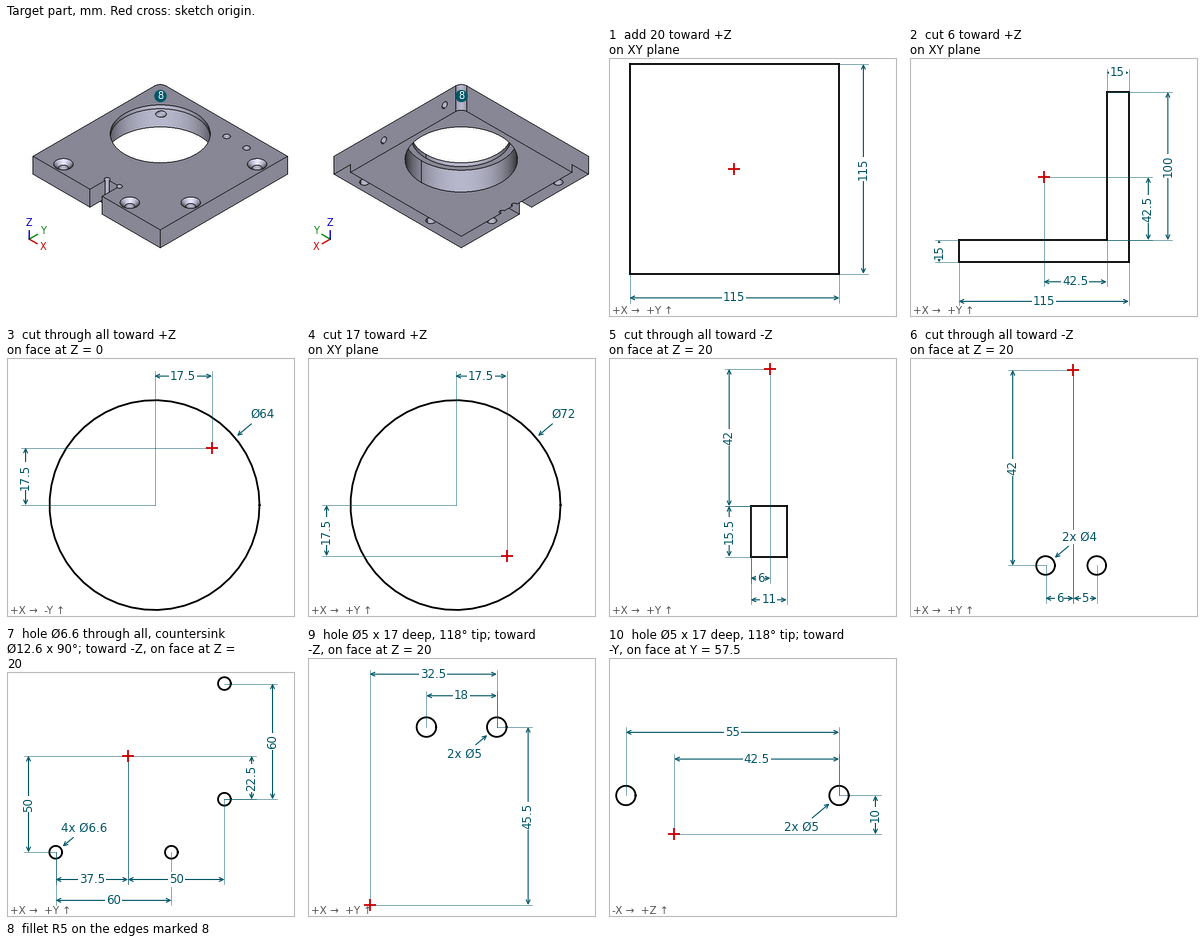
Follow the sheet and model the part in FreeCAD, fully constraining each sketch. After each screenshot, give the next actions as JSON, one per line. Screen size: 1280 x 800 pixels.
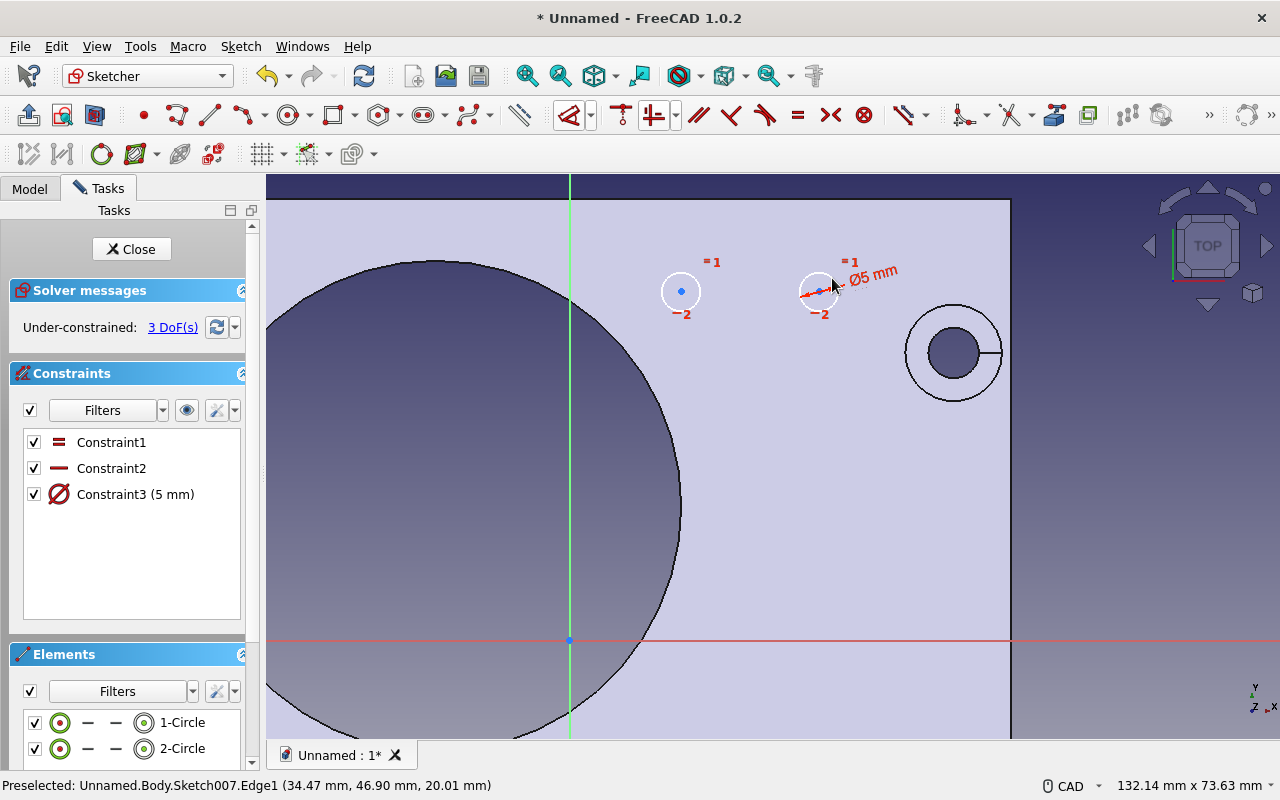
{"action": "left_click", "coordinate": [819, 292]}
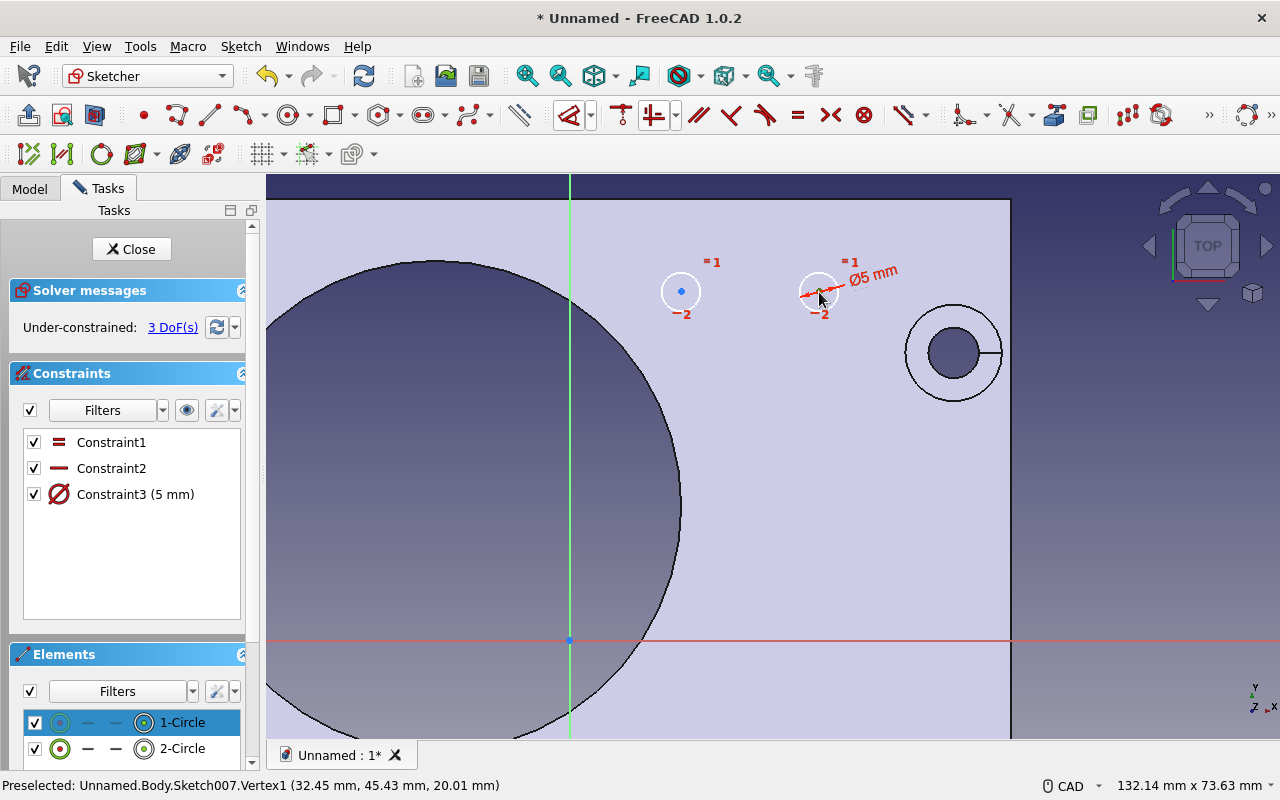
{"action": "left_click", "coordinate": [681, 292]}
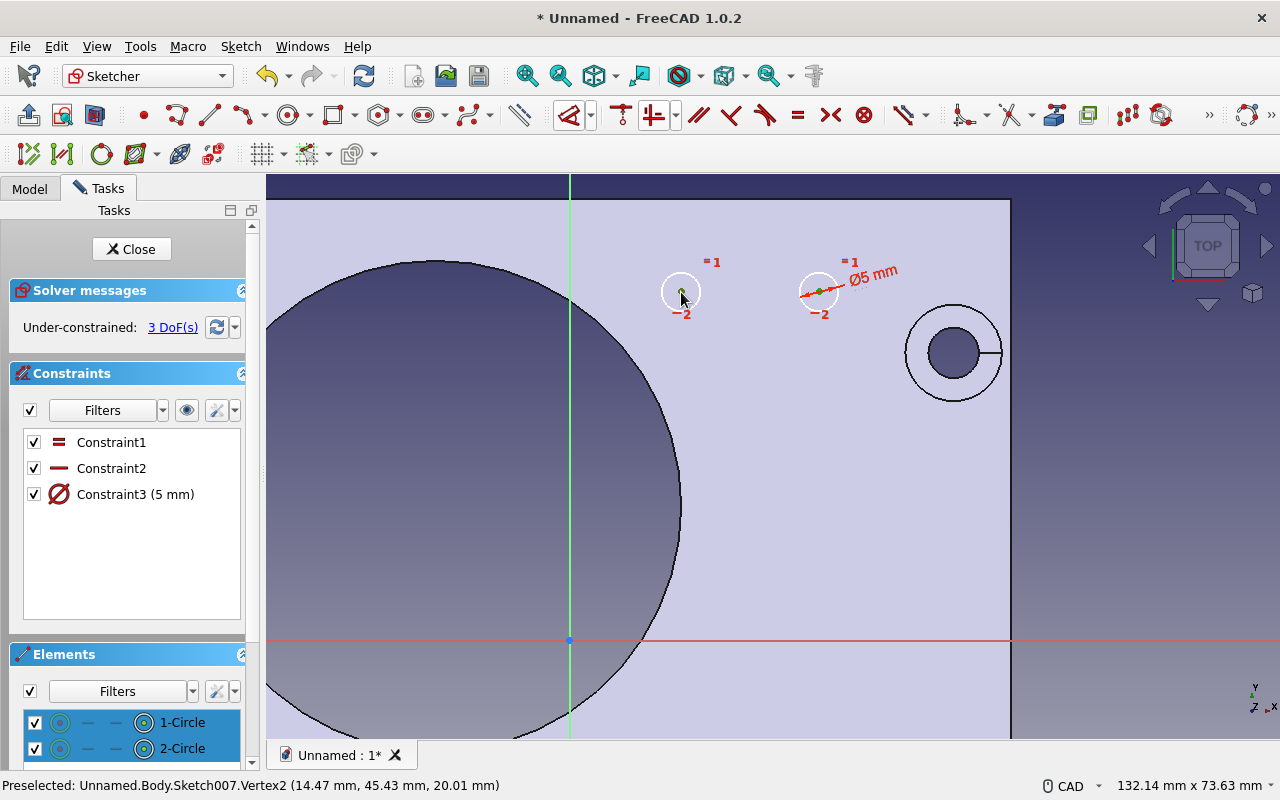
{"action": "key", "text": "l"}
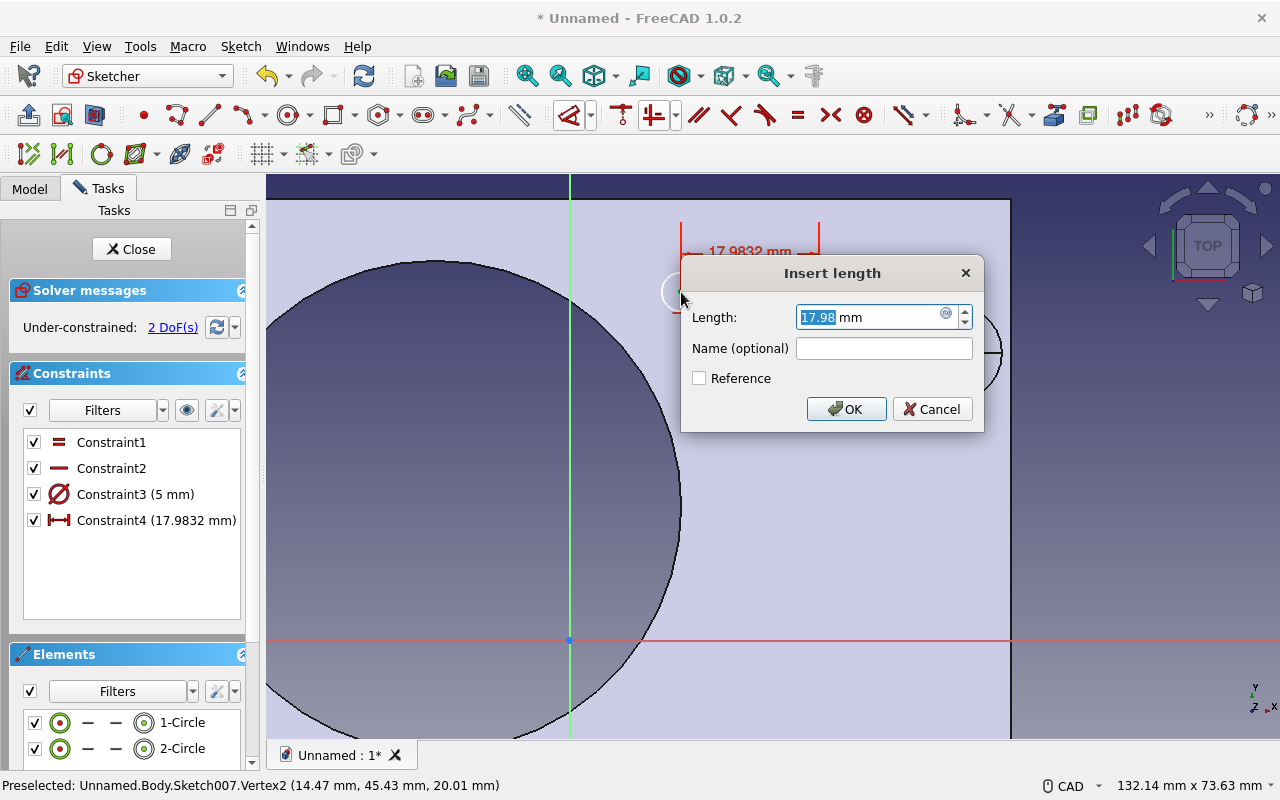
{"action": "type", "text": "18"}
{"action": "key", "text": "Return"}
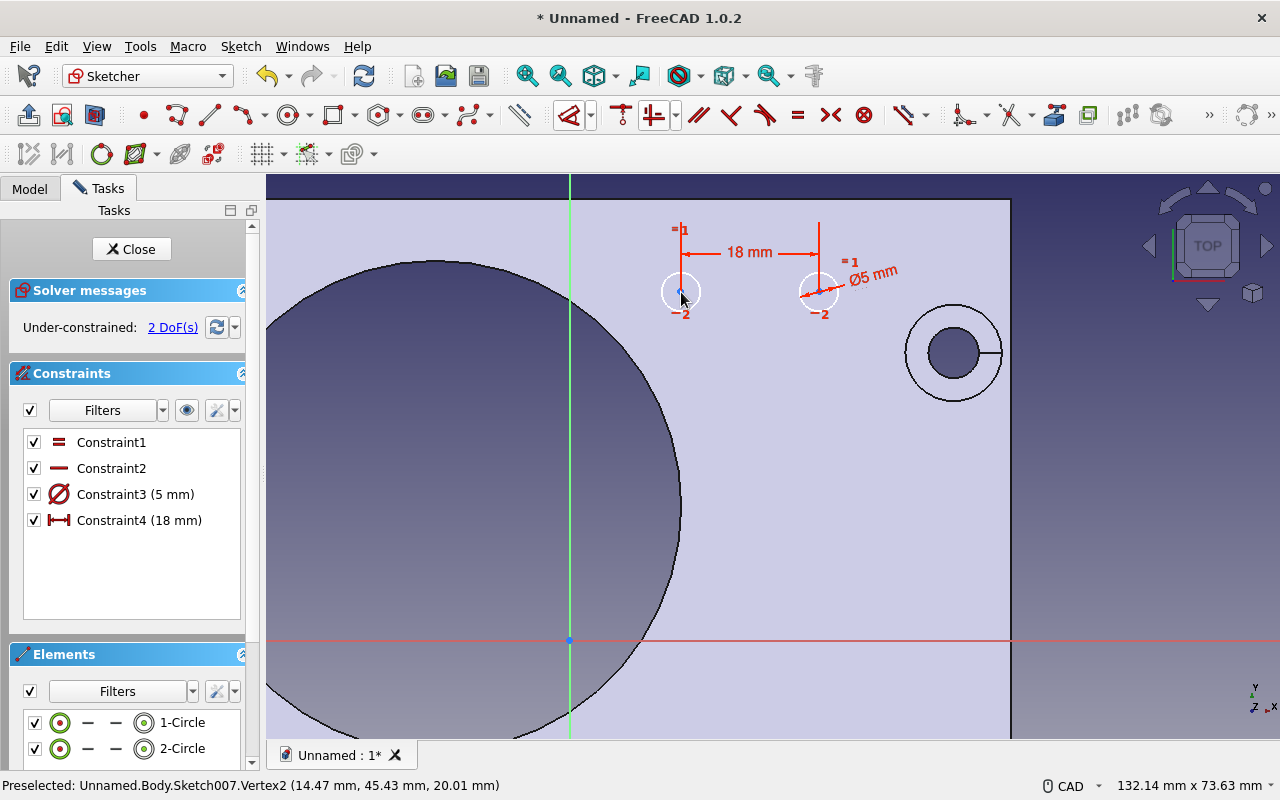
{"action": "left_click", "coordinate": [819, 292]}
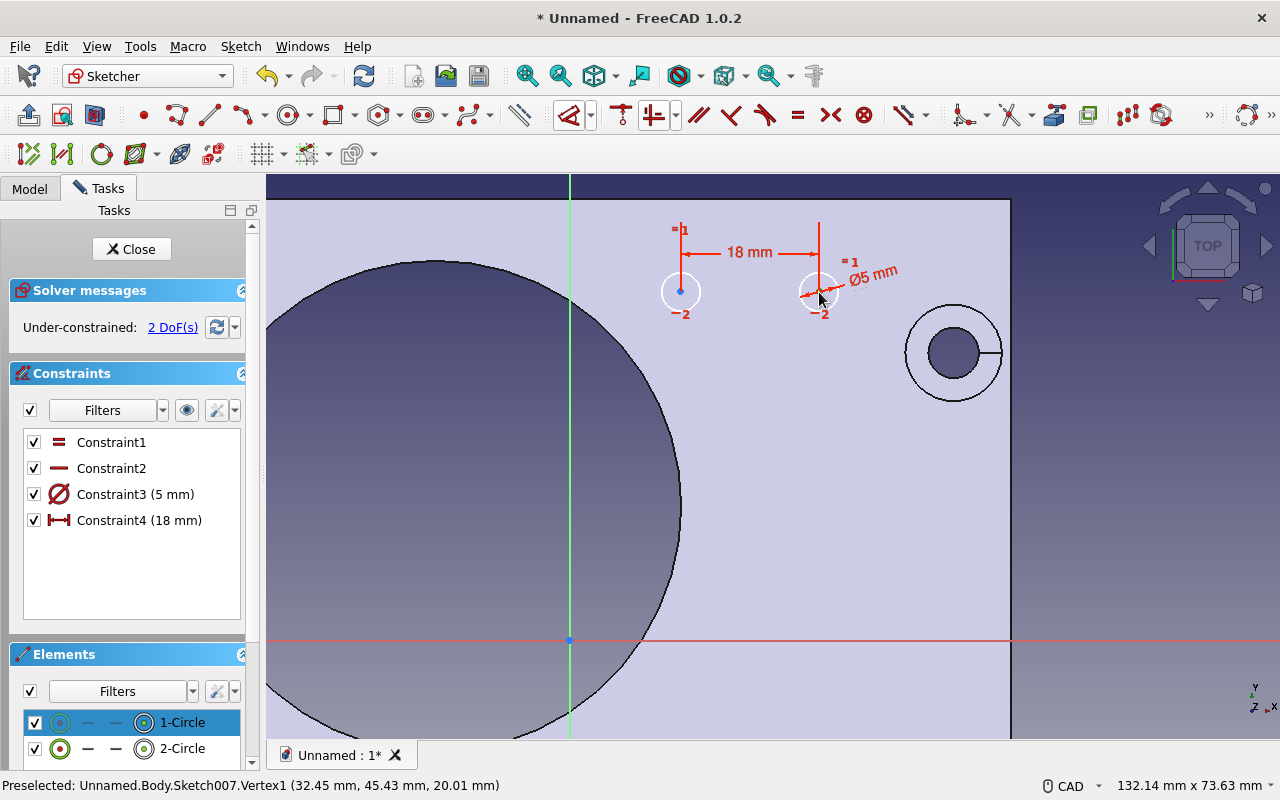
{"action": "key", "text": "l"}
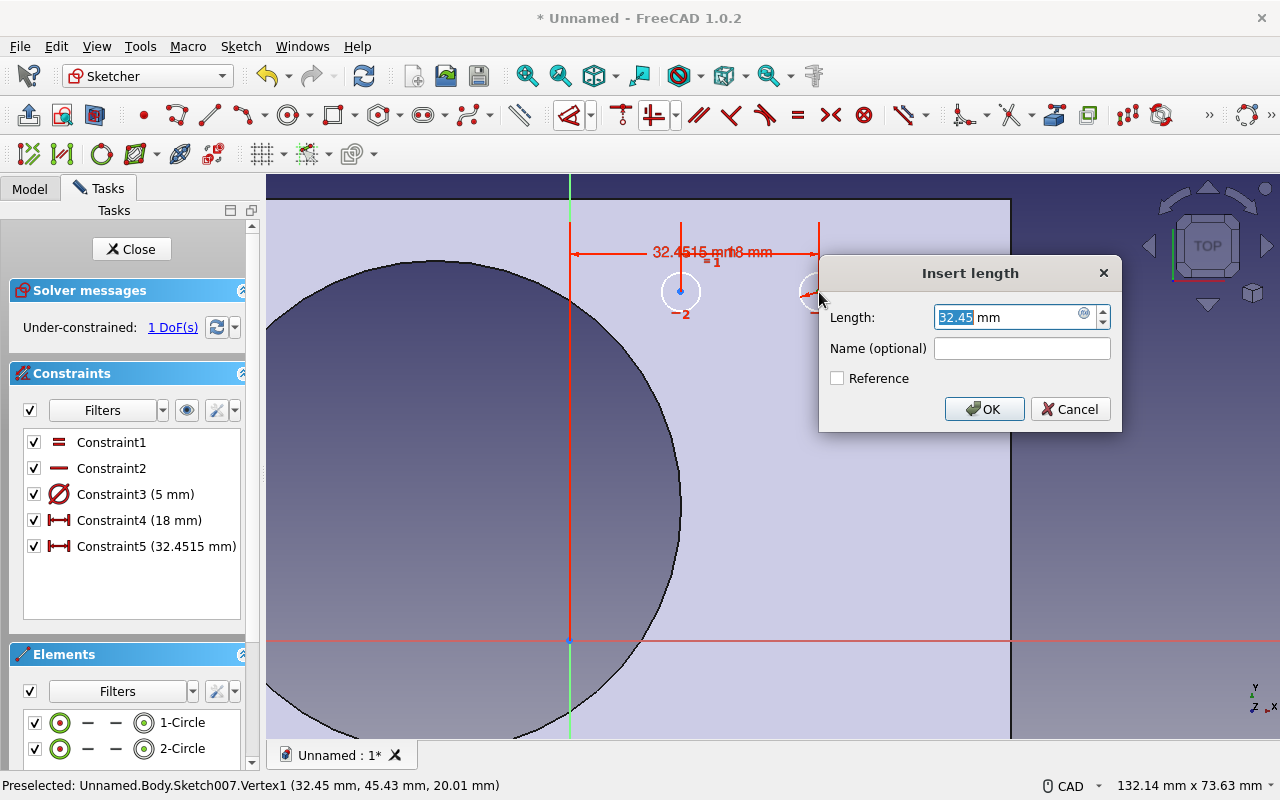
{"action": "type", "text": "32.5"}
{"action": "key", "text": "Return"}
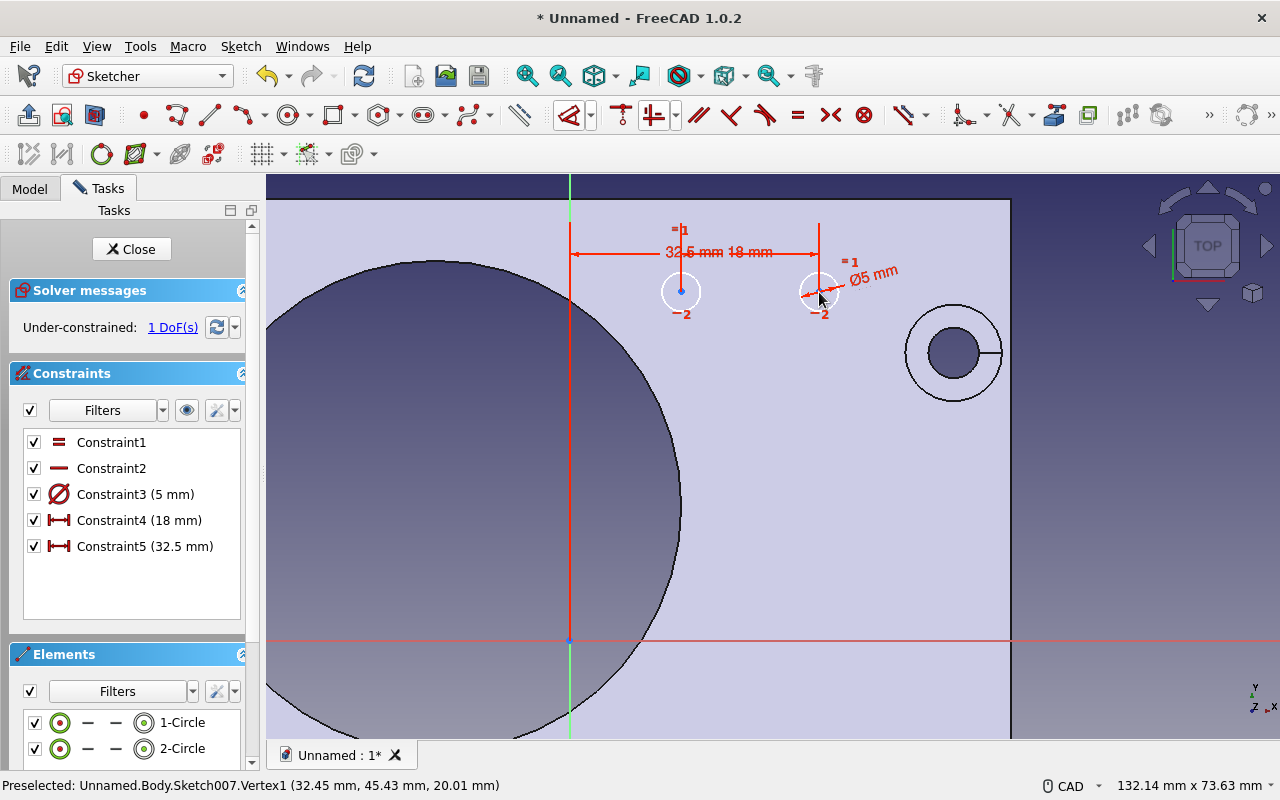
{"action": "left_click", "coordinate": [819, 292]}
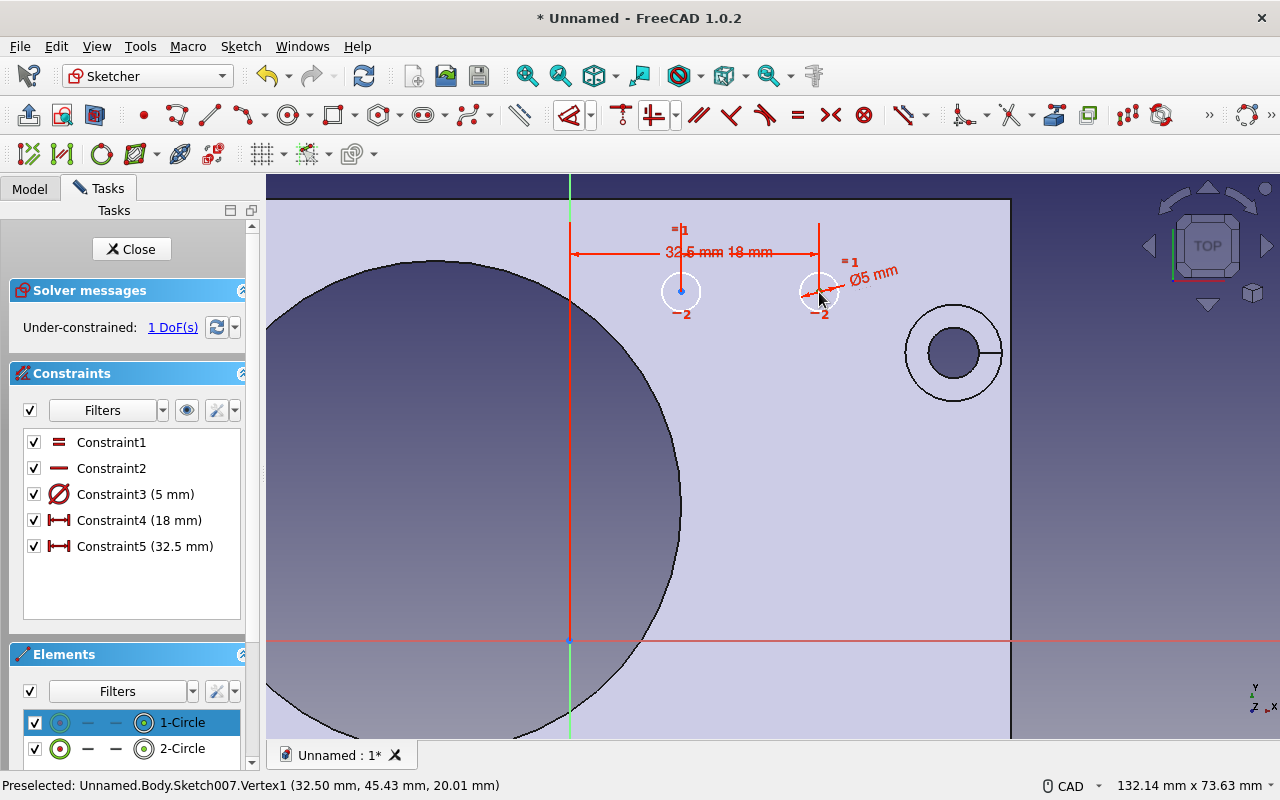
{"action": "key", "text": "i"}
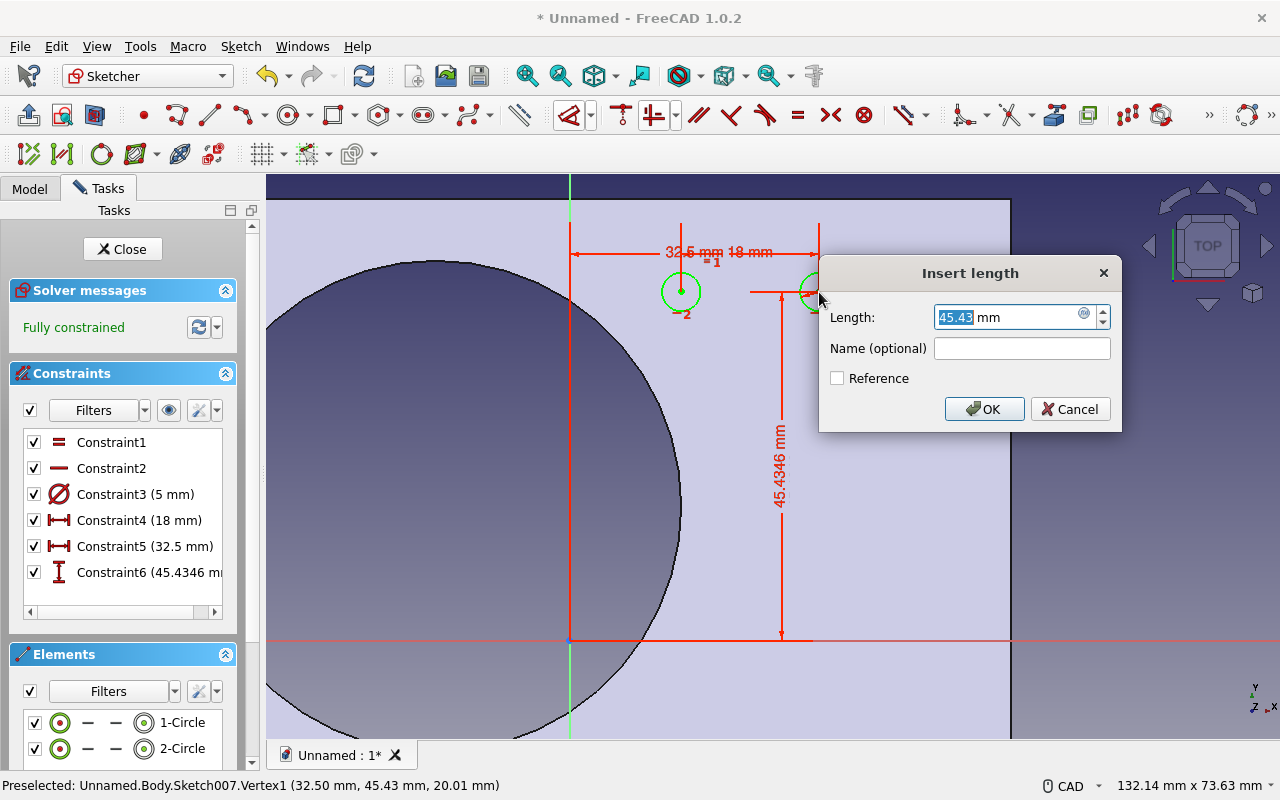
{"action": "type", "text": "45.5"}
{"action": "key", "text": "Return"}